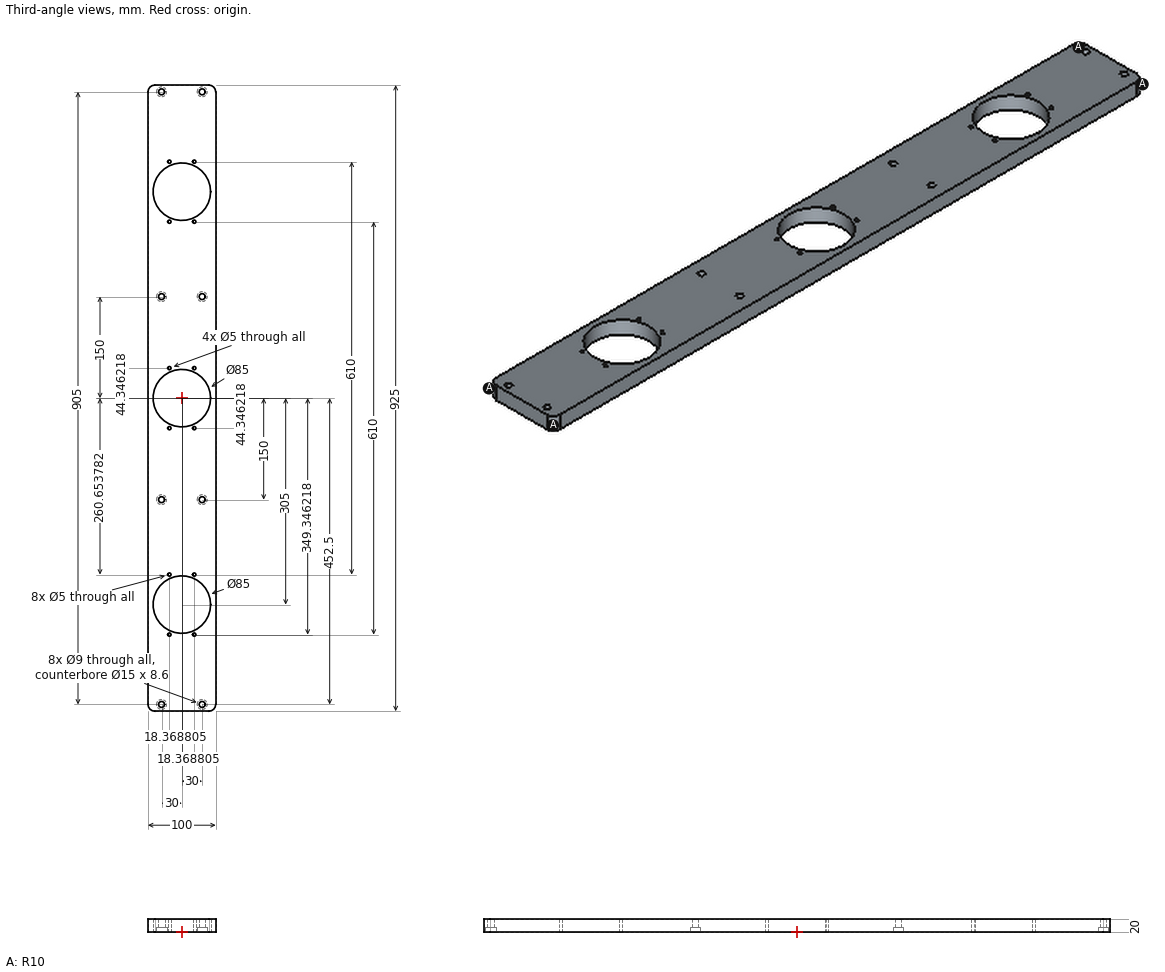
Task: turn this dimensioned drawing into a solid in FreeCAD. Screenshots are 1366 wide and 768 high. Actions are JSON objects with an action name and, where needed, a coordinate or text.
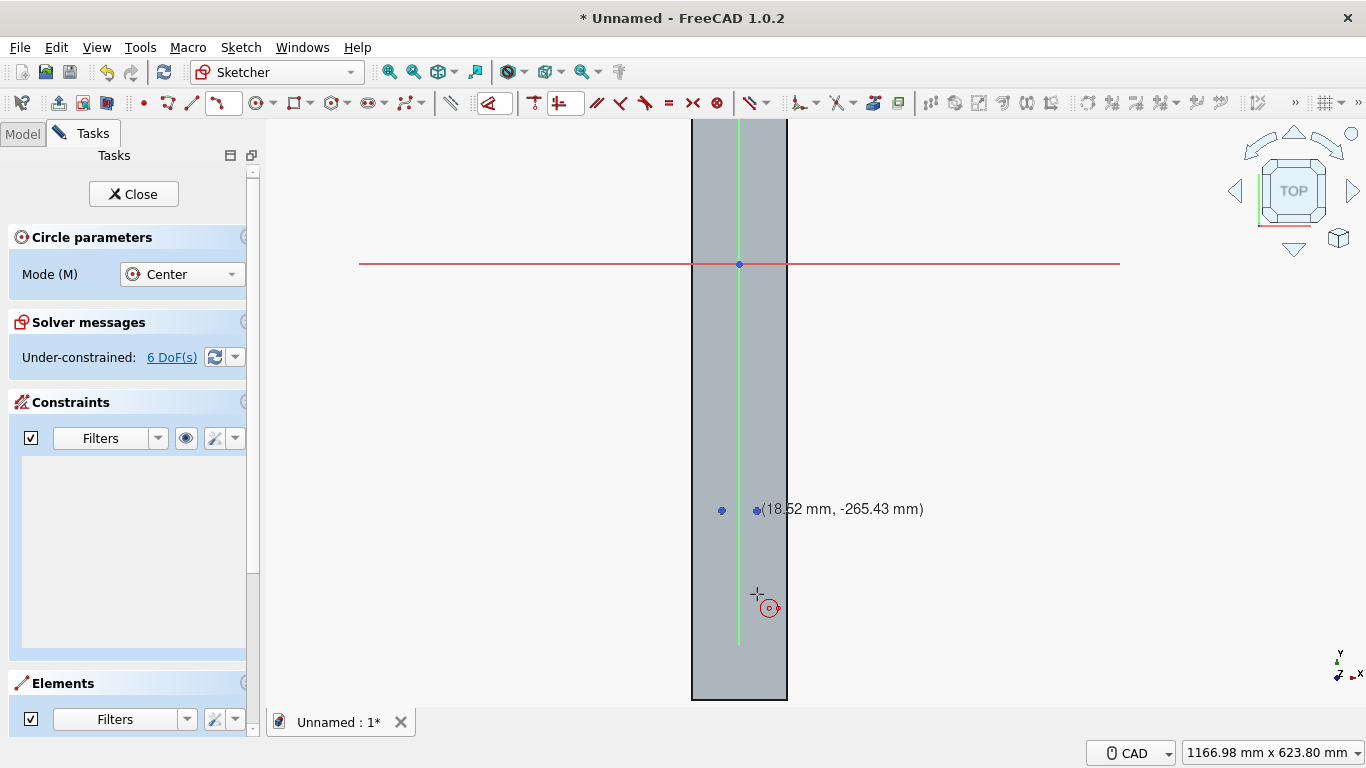
{"action": "left_click", "coordinate": [757, 593]}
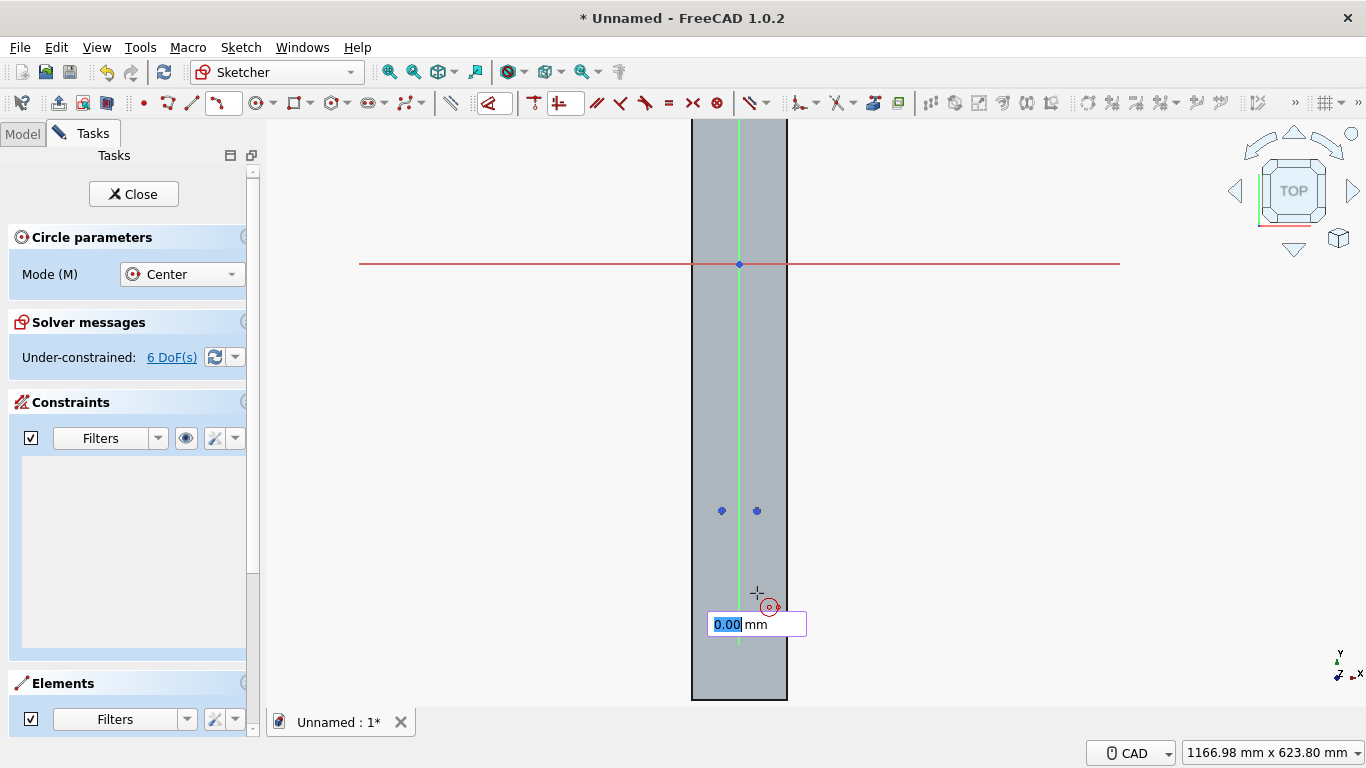
{"action": "scroll", "coordinate": [758, 592], "scroll_direction": "up", "scroll_amount": 10}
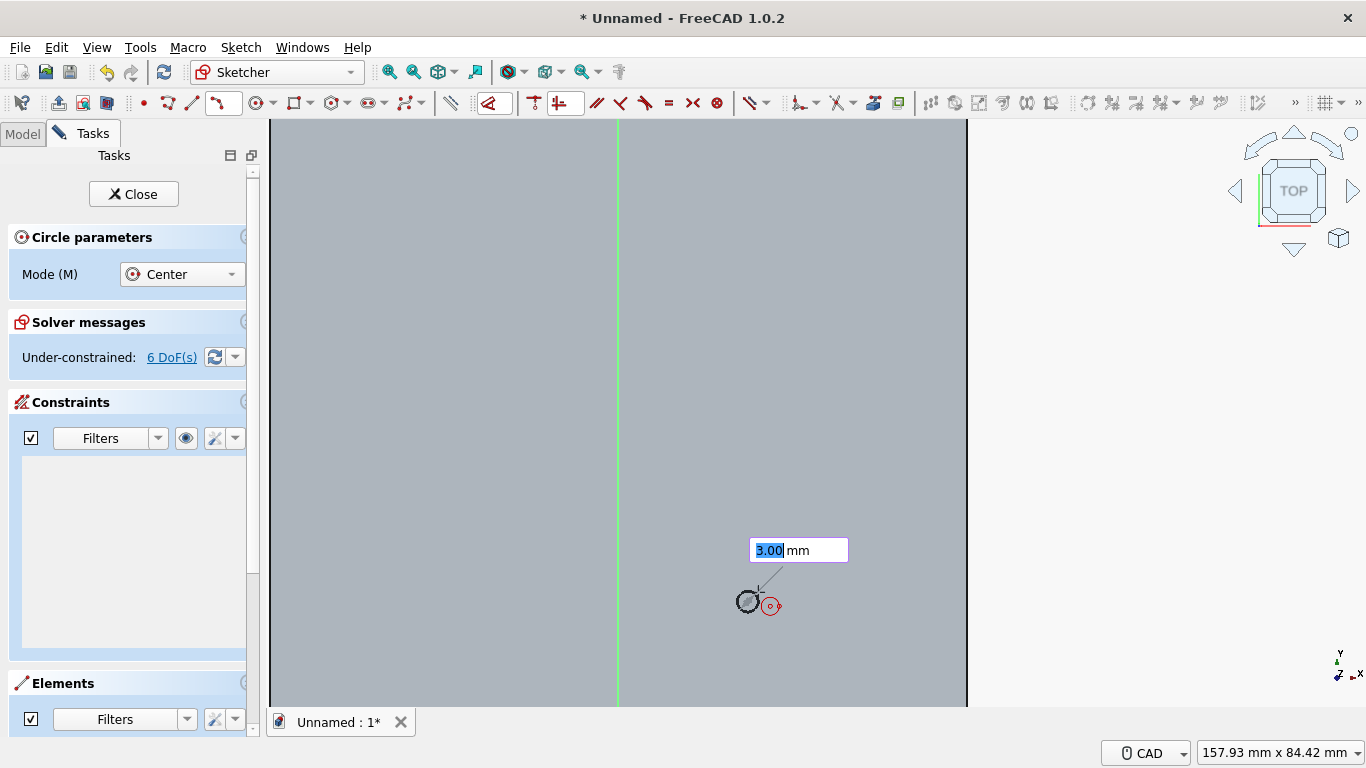
{"action": "left_click", "coordinate": [759, 585]}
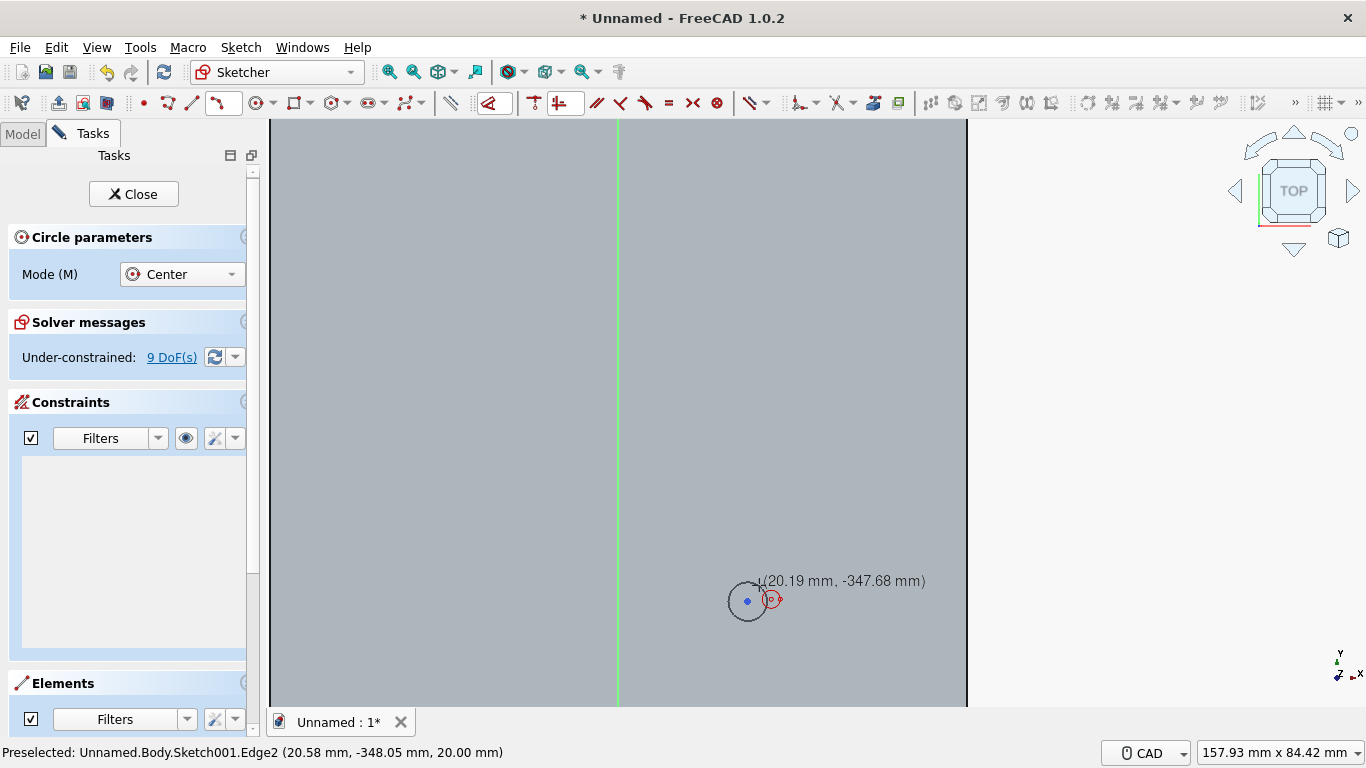
{"action": "scroll", "coordinate": [490, 598], "scroll_direction": "up", "scroll_amount": 2}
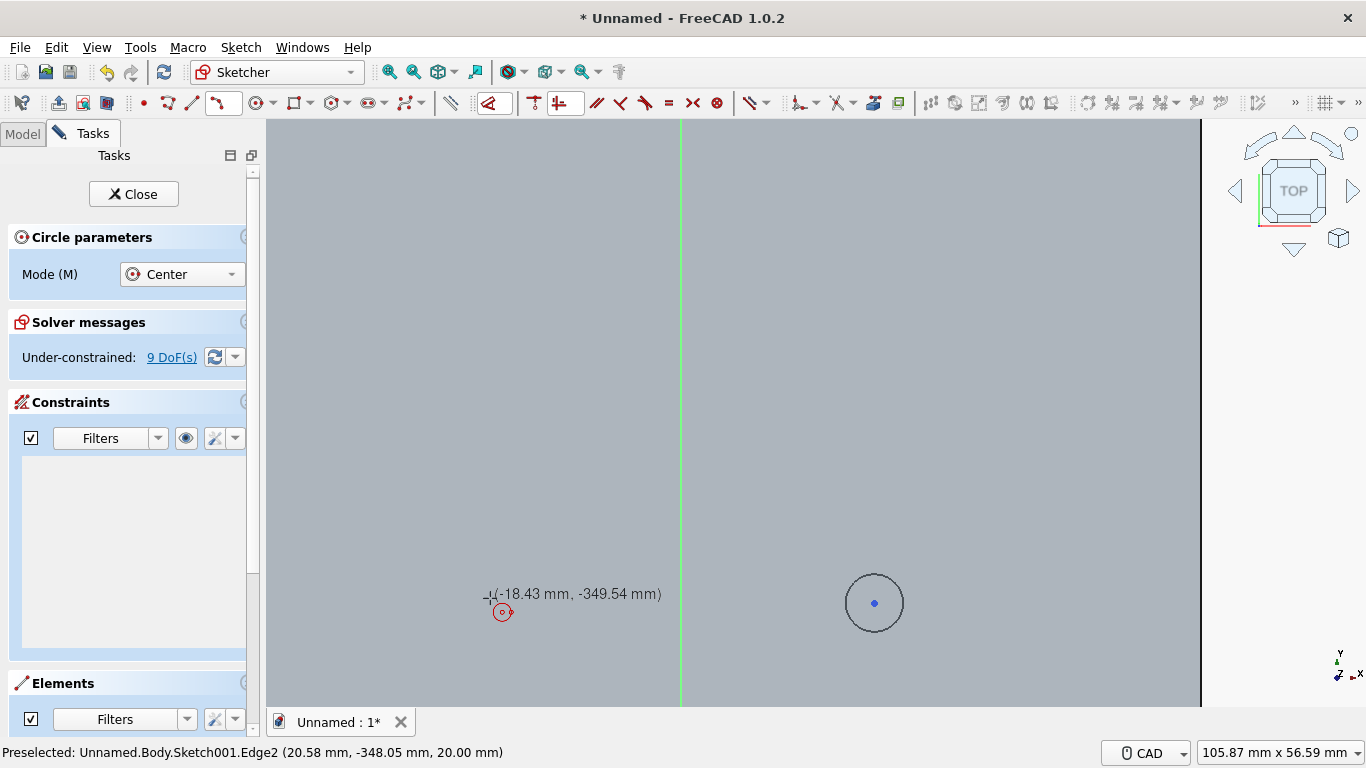
{"action": "scroll", "coordinate": [751, 594], "scroll_direction": "down", "scroll_amount": 15}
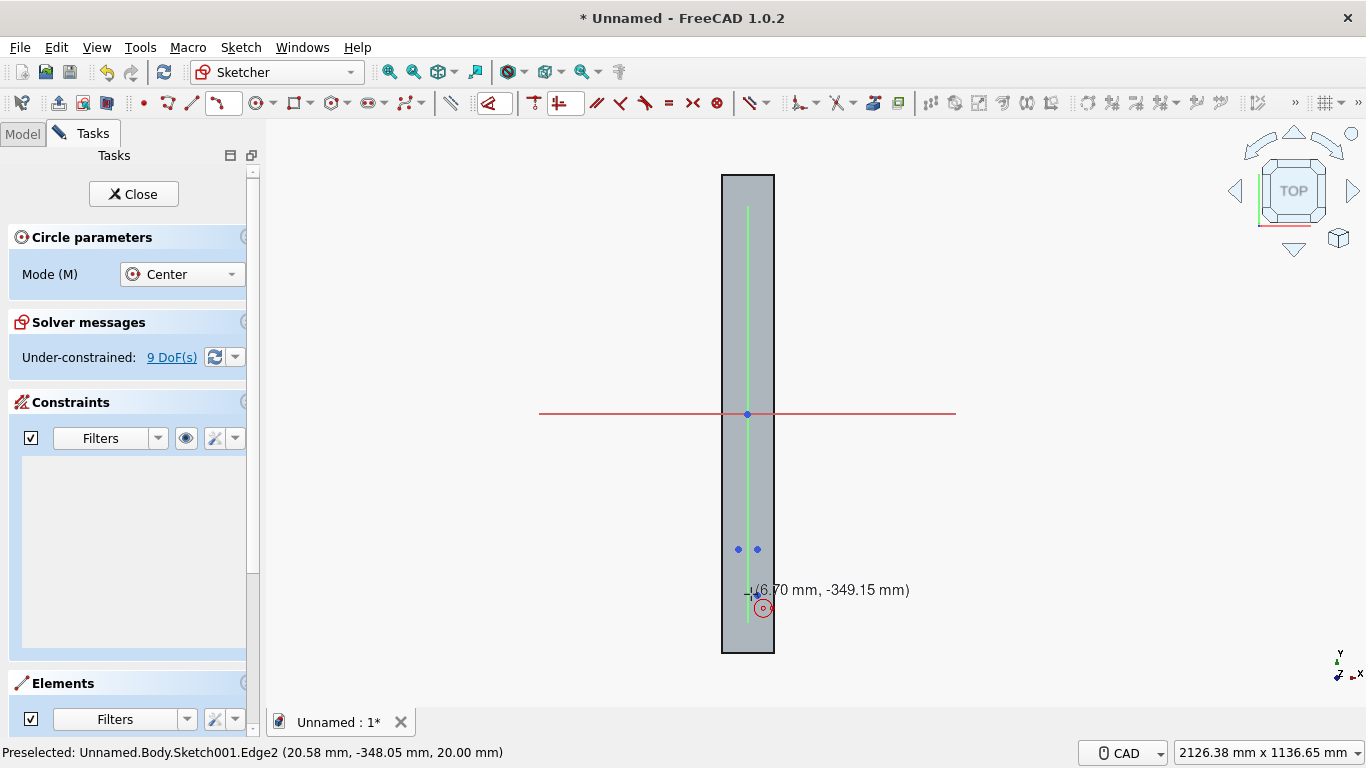
{"action": "scroll", "coordinate": [738, 595], "scroll_direction": "up", "scroll_amount": 3}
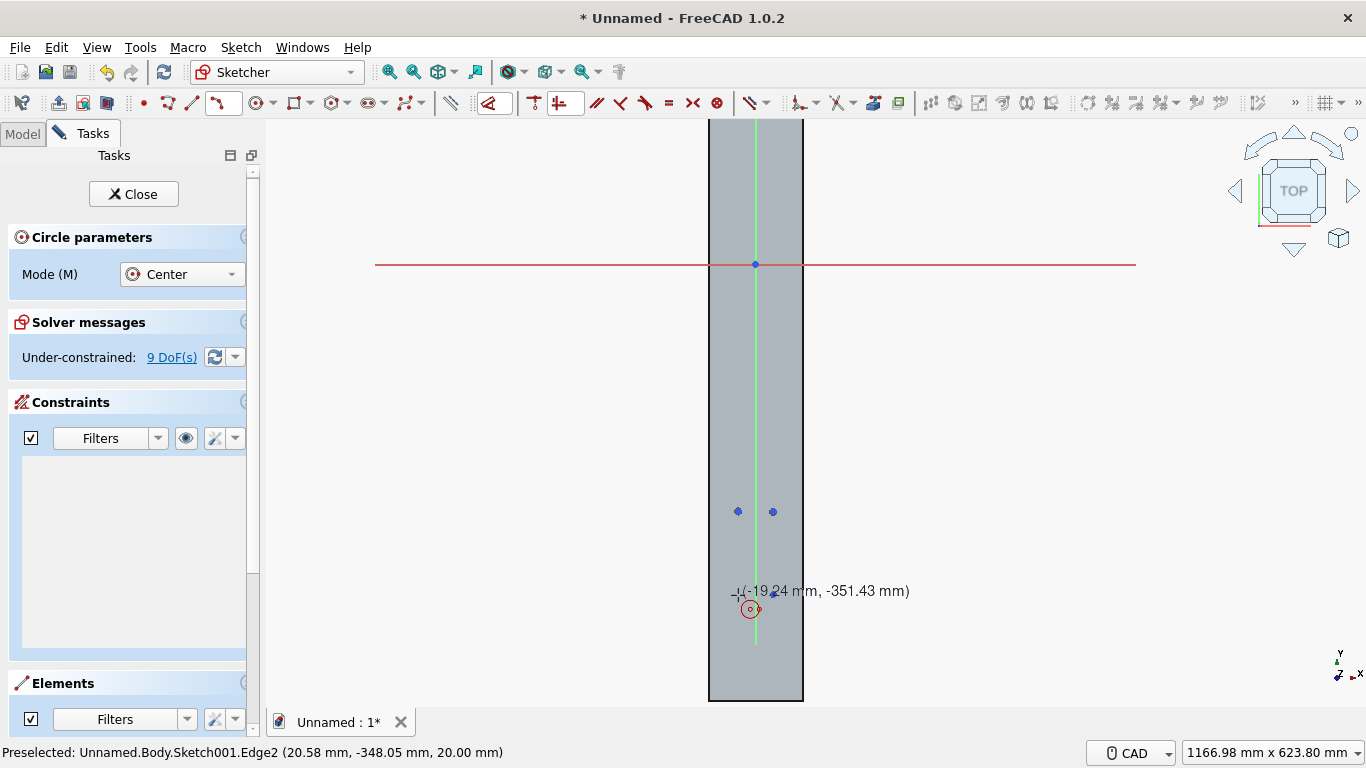
{"action": "left_click", "coordinate": [738, 594]}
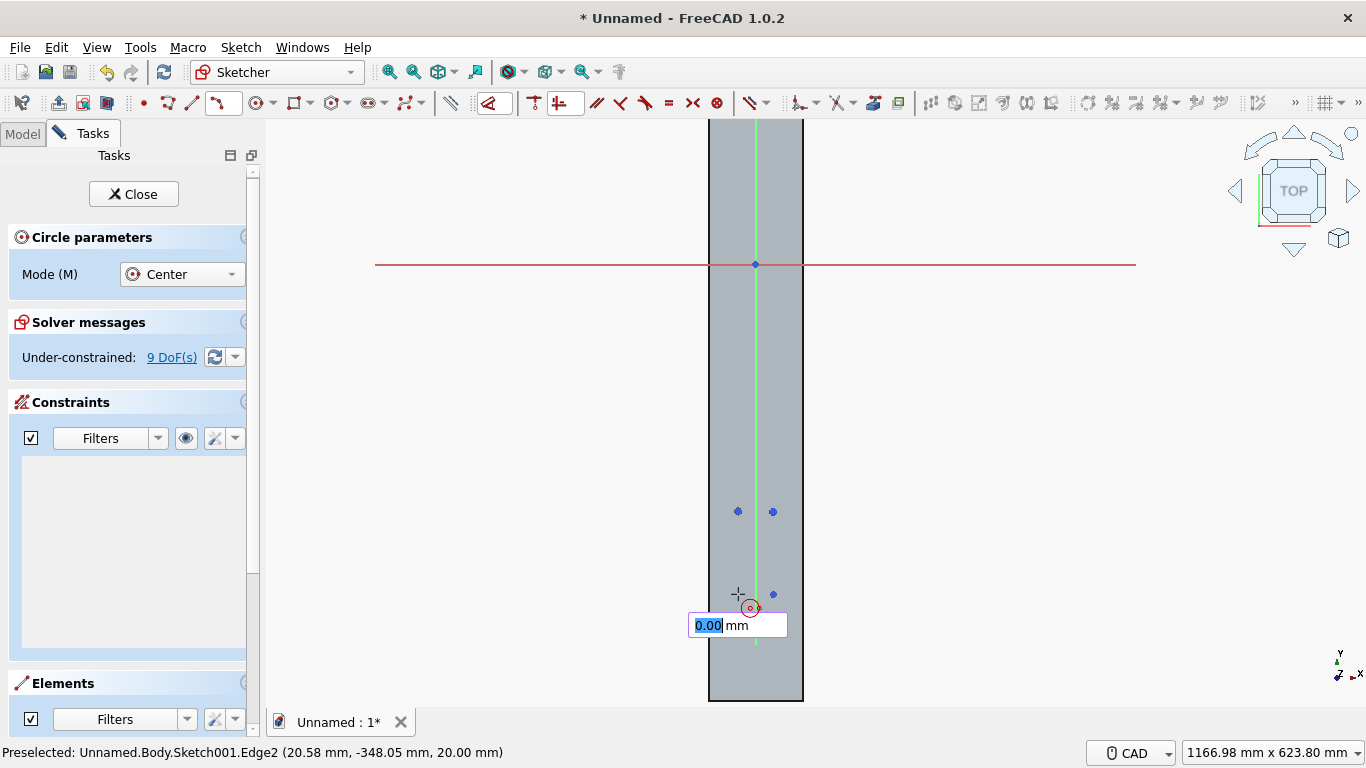
{"action": "scroll", "coordinate": [740, 593], "scroll_direction": "up", "scroll_amount": 10}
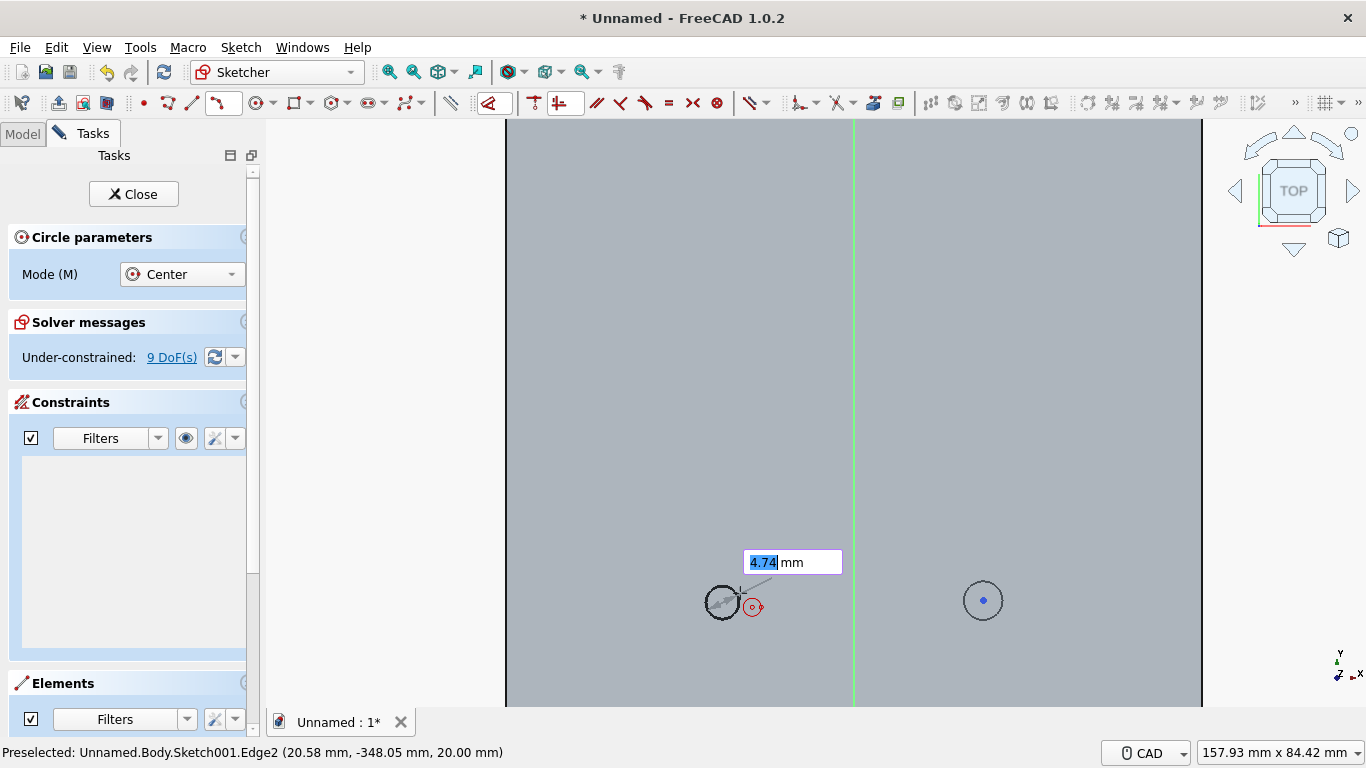
{"action": "left_click", "coordinate": [738, 584]}